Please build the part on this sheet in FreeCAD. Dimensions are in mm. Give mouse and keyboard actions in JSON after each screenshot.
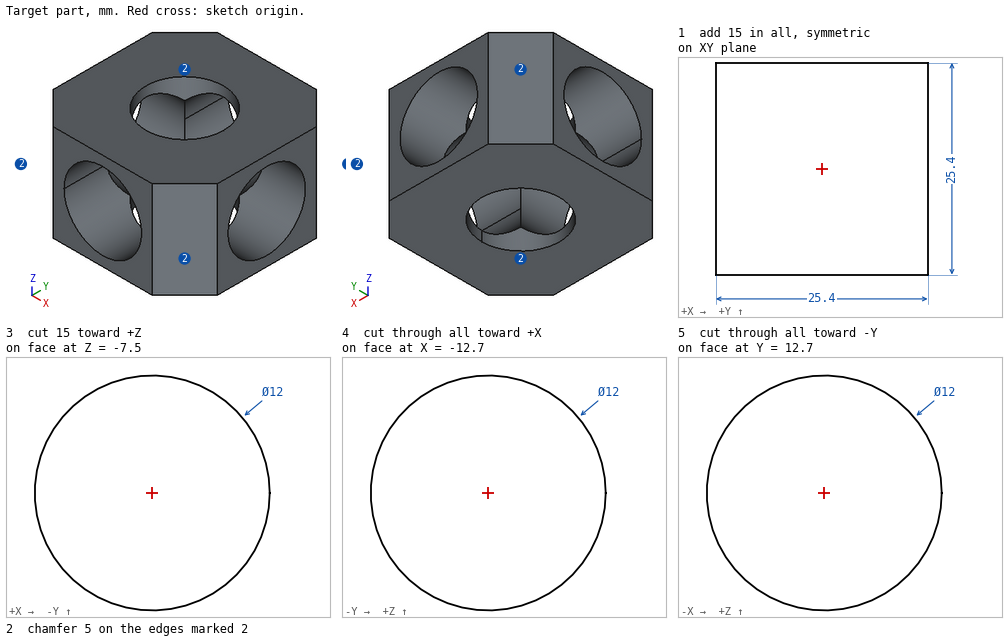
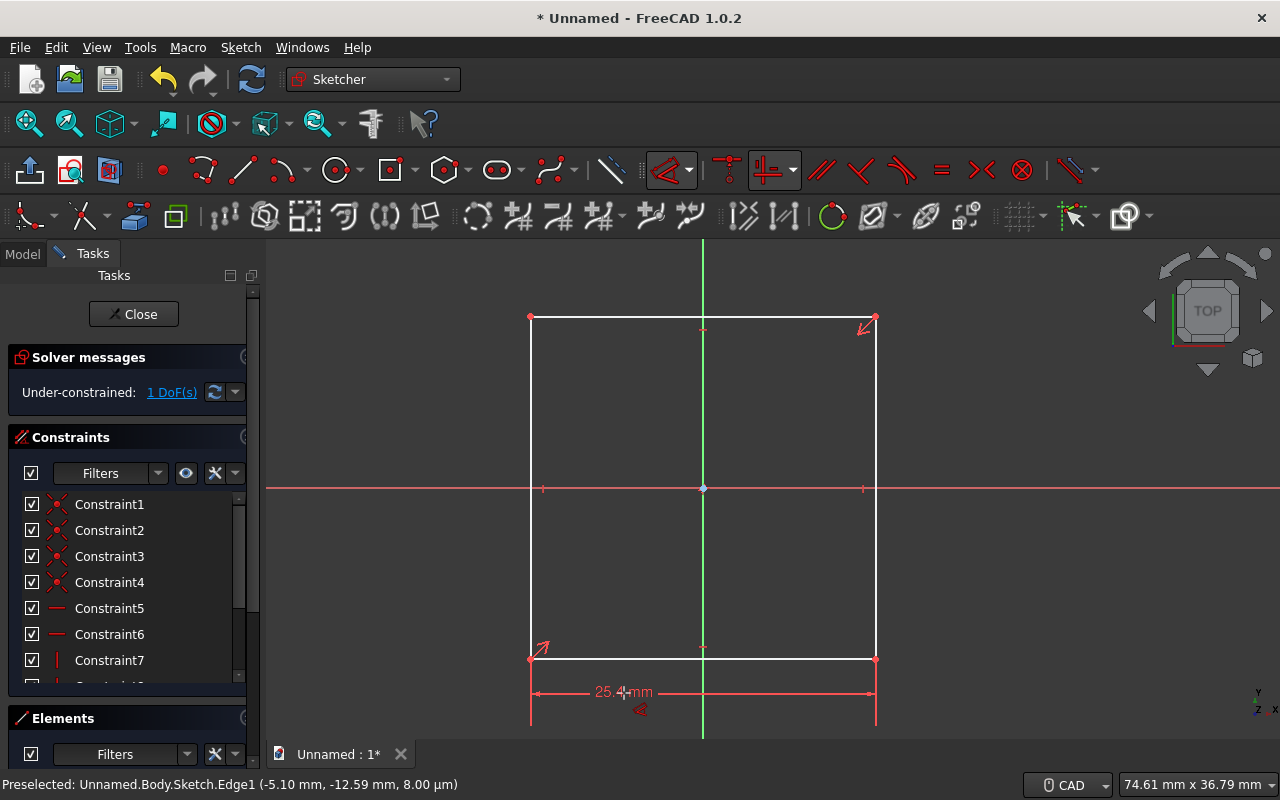
{"action": "left_click", "coordinate": [876, 557]}
{"action": "left_click", "coordinate": [910, 409]}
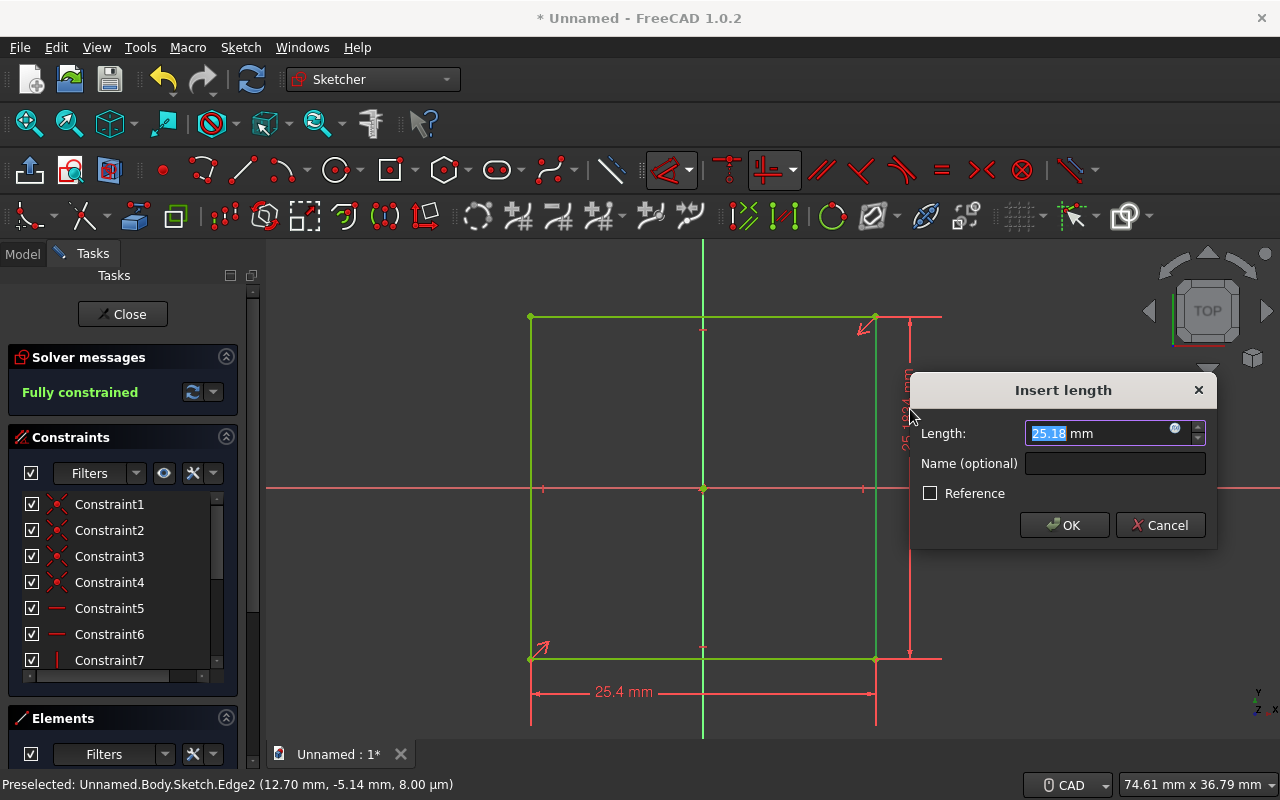
{"action": "type", "text": "25.4"}
{"action": "key", "text": "Return"}
{"action": "key", "text": "Escape"}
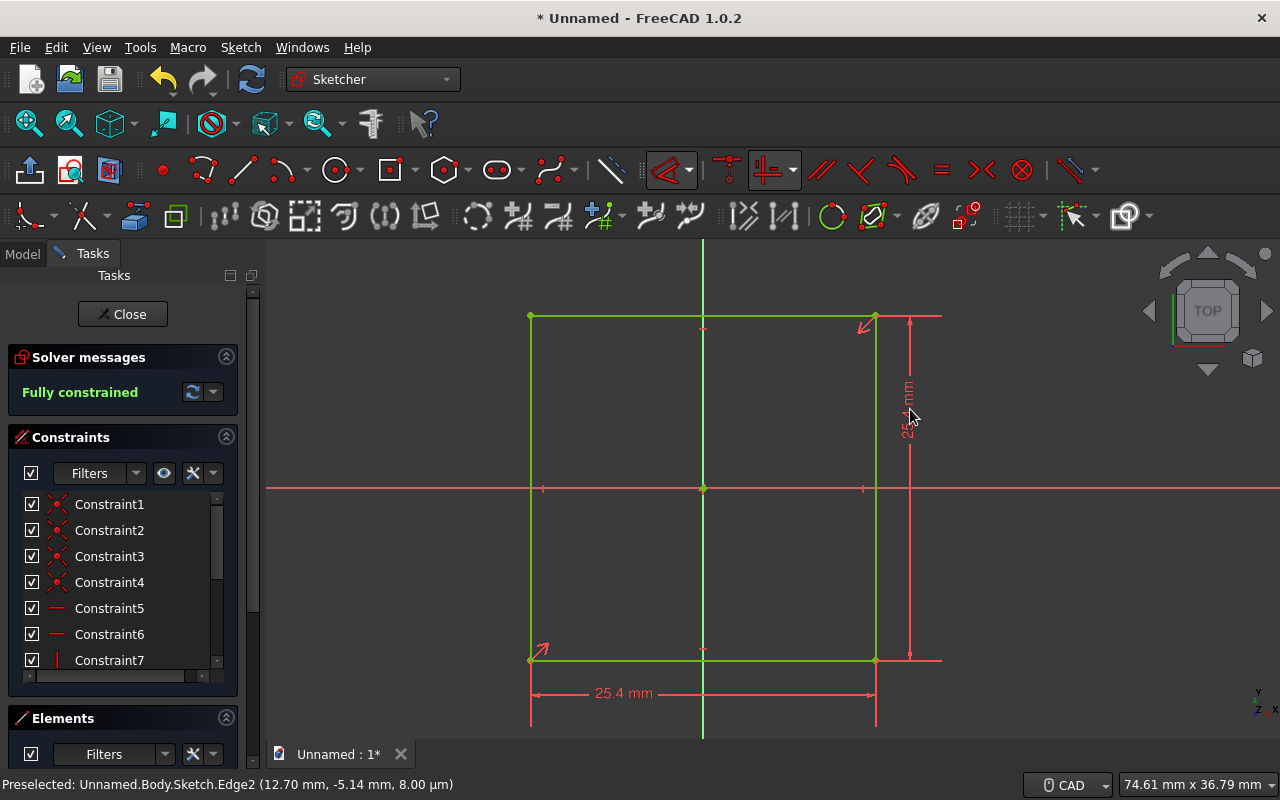
{"action": "left_click", "coordinate": [123, 314]}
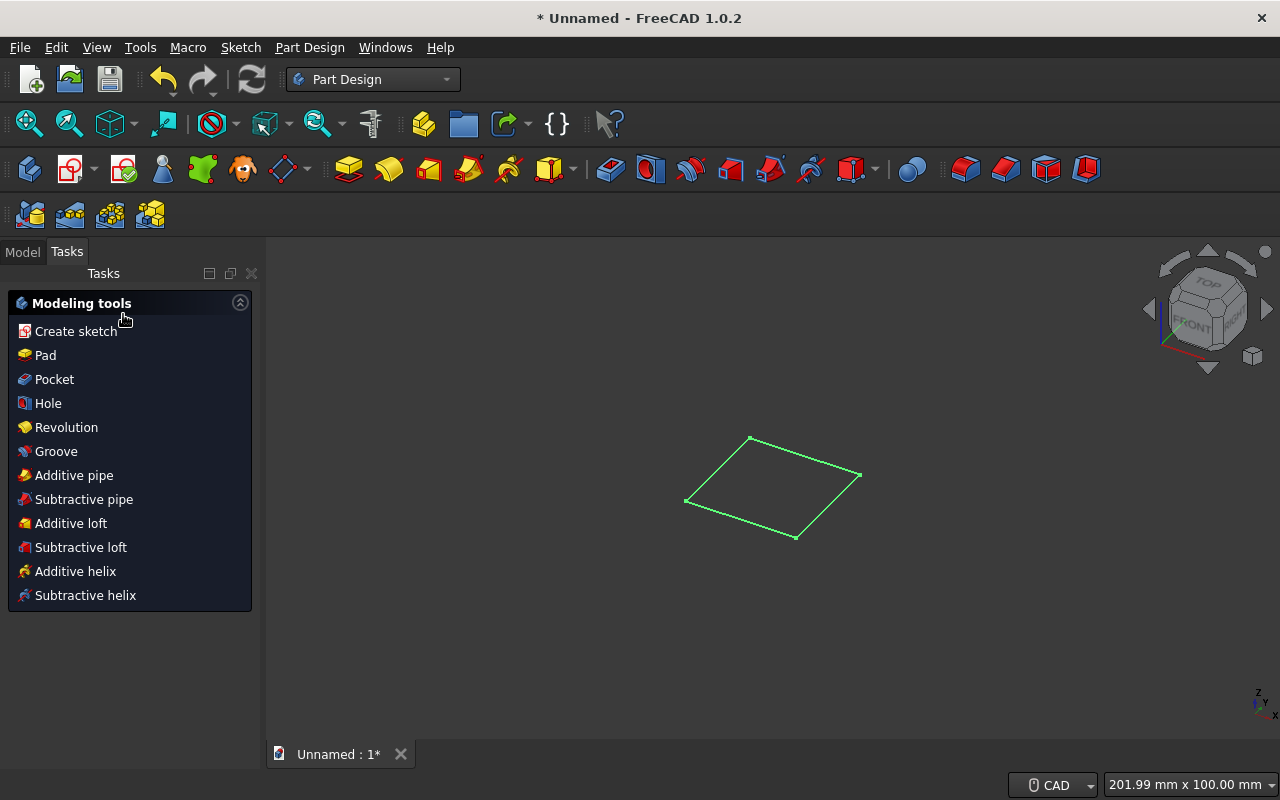
{"action": "left_click", "coordinate": [350, 170]}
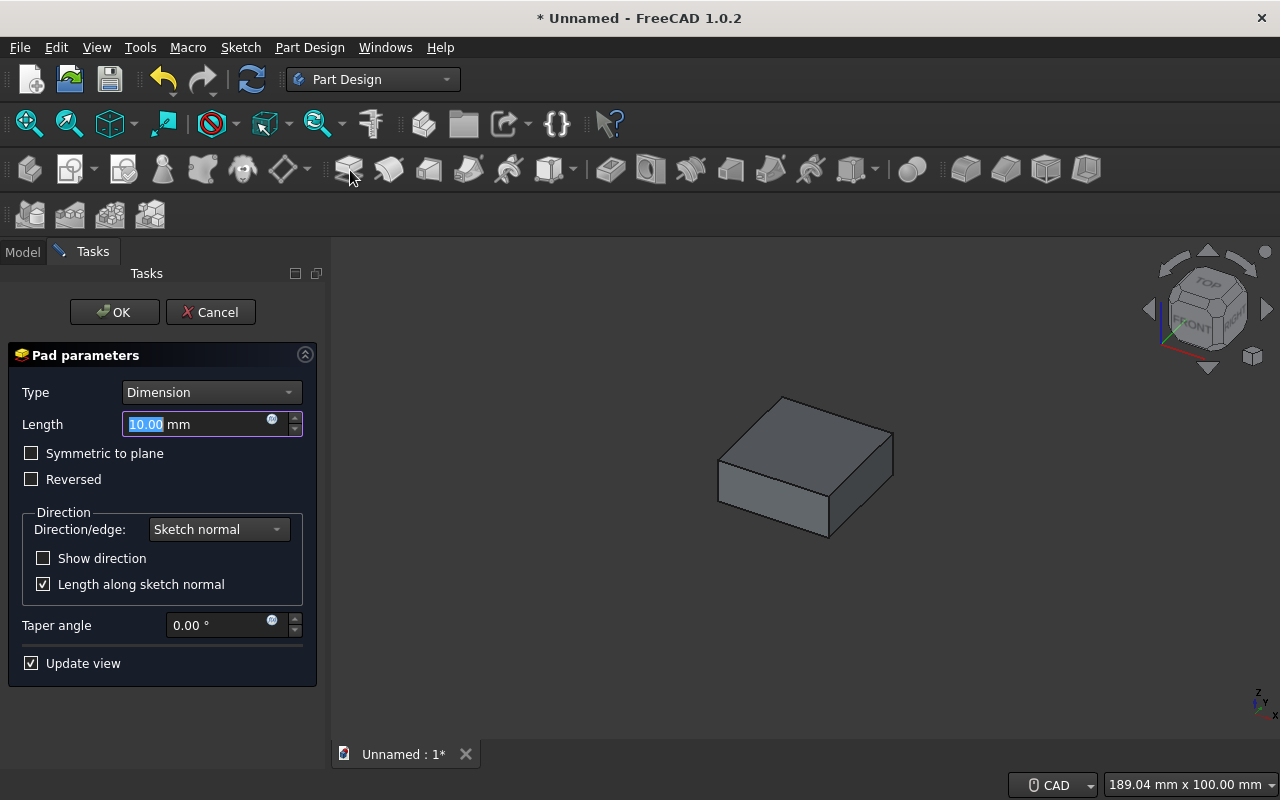
{"action": "type", "text": "15"}
{"action": "key", "text": "Tab"}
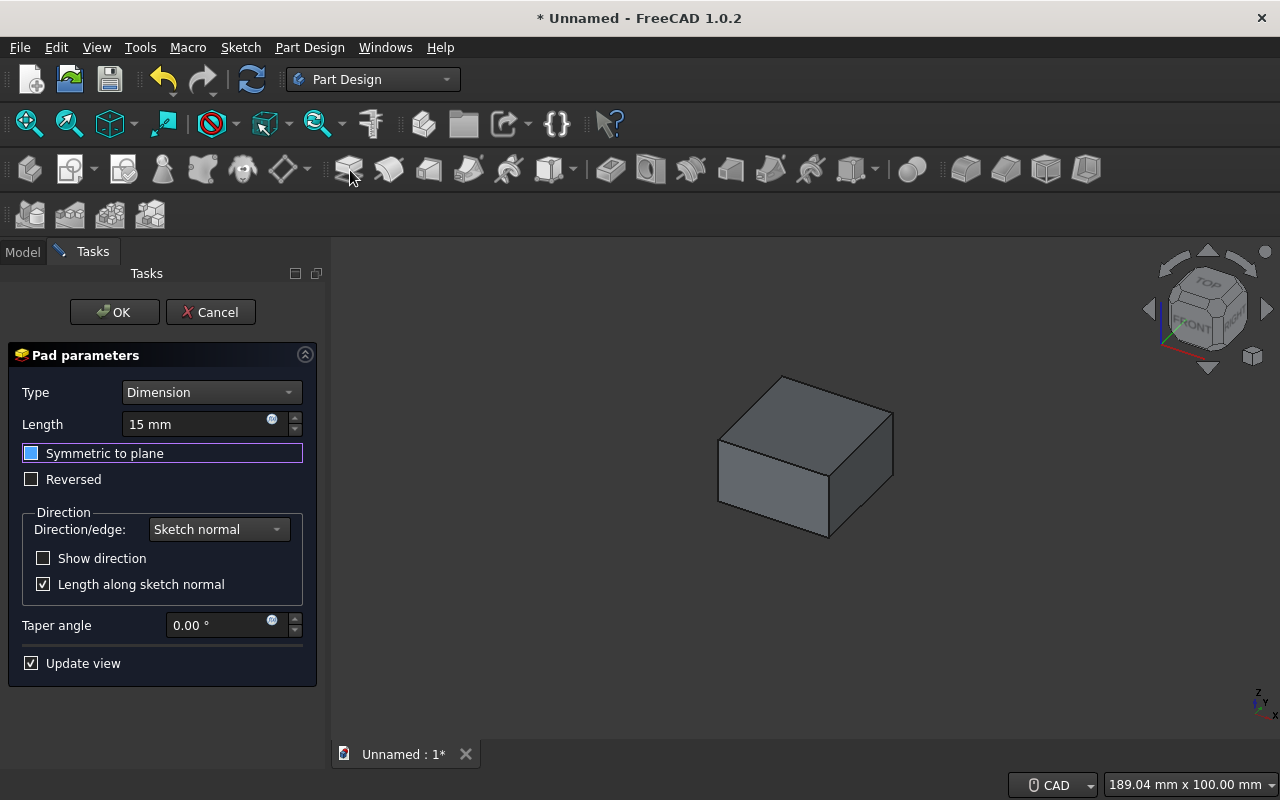
{"action": "left_click", "coordinate": [30, 453]}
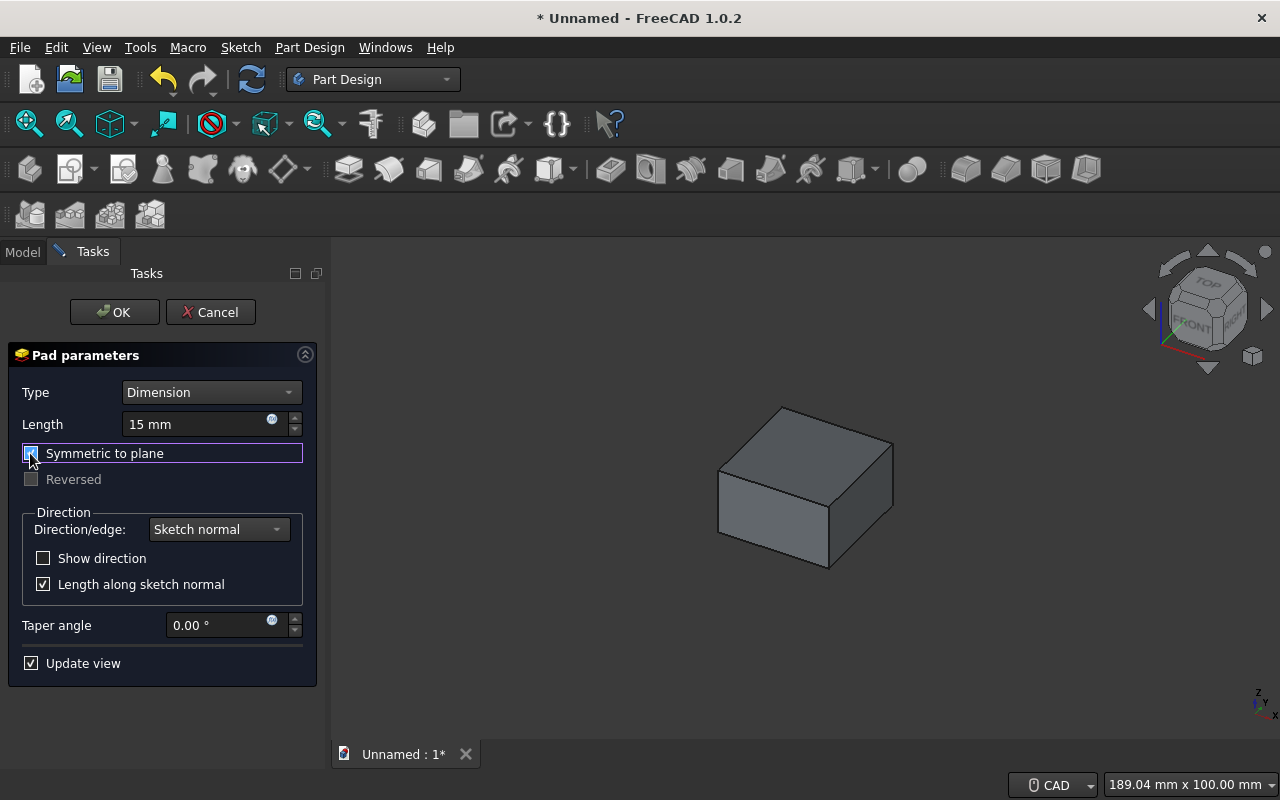
{"action": "left_click", "coordinate": [115, 312]}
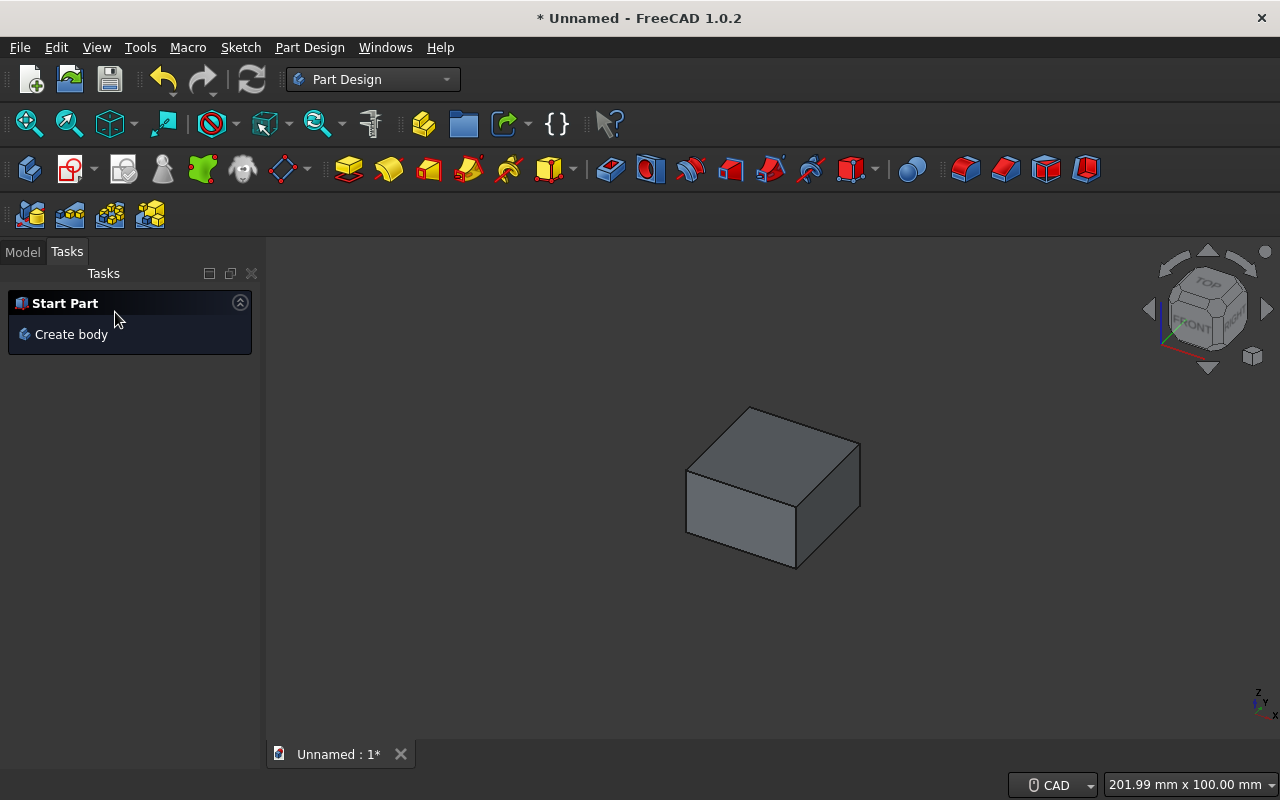
{"action": "key", "text": "v f"}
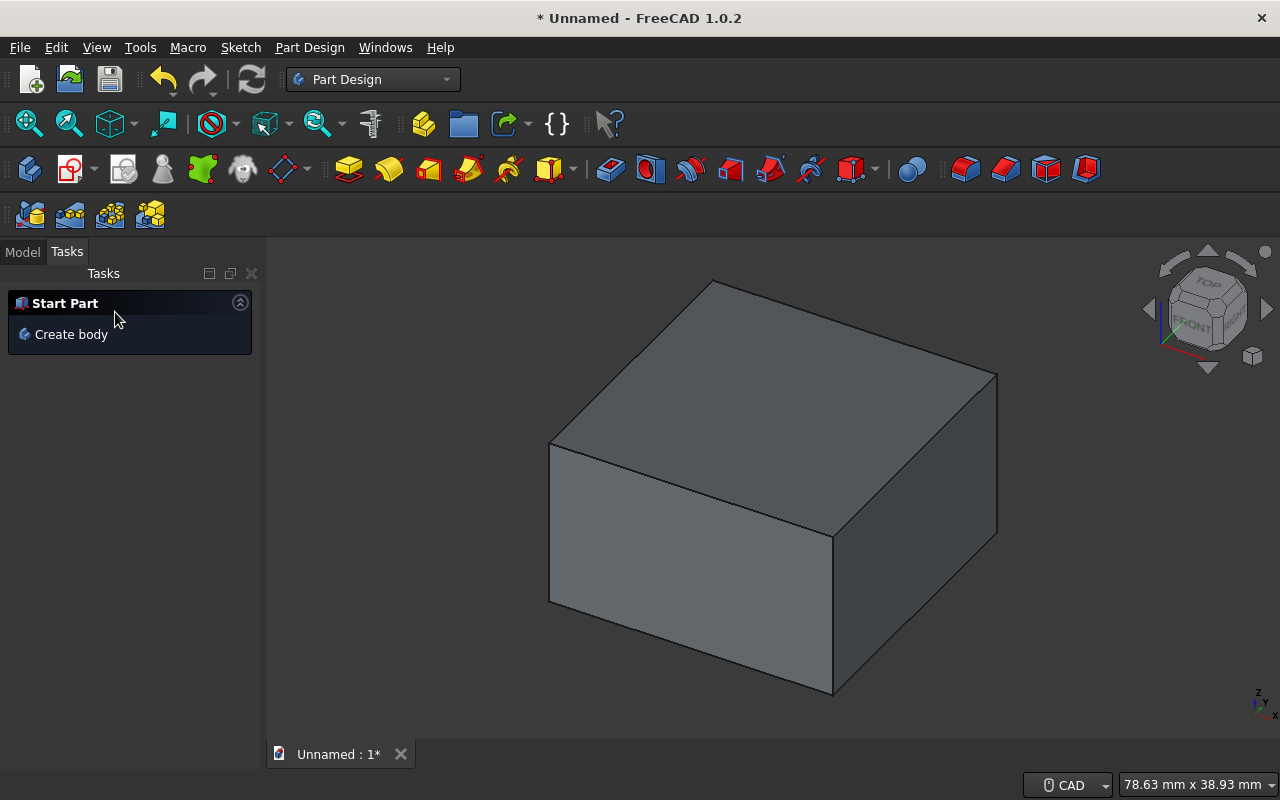
{"action": "left_click", "coordinate": [833, 615]}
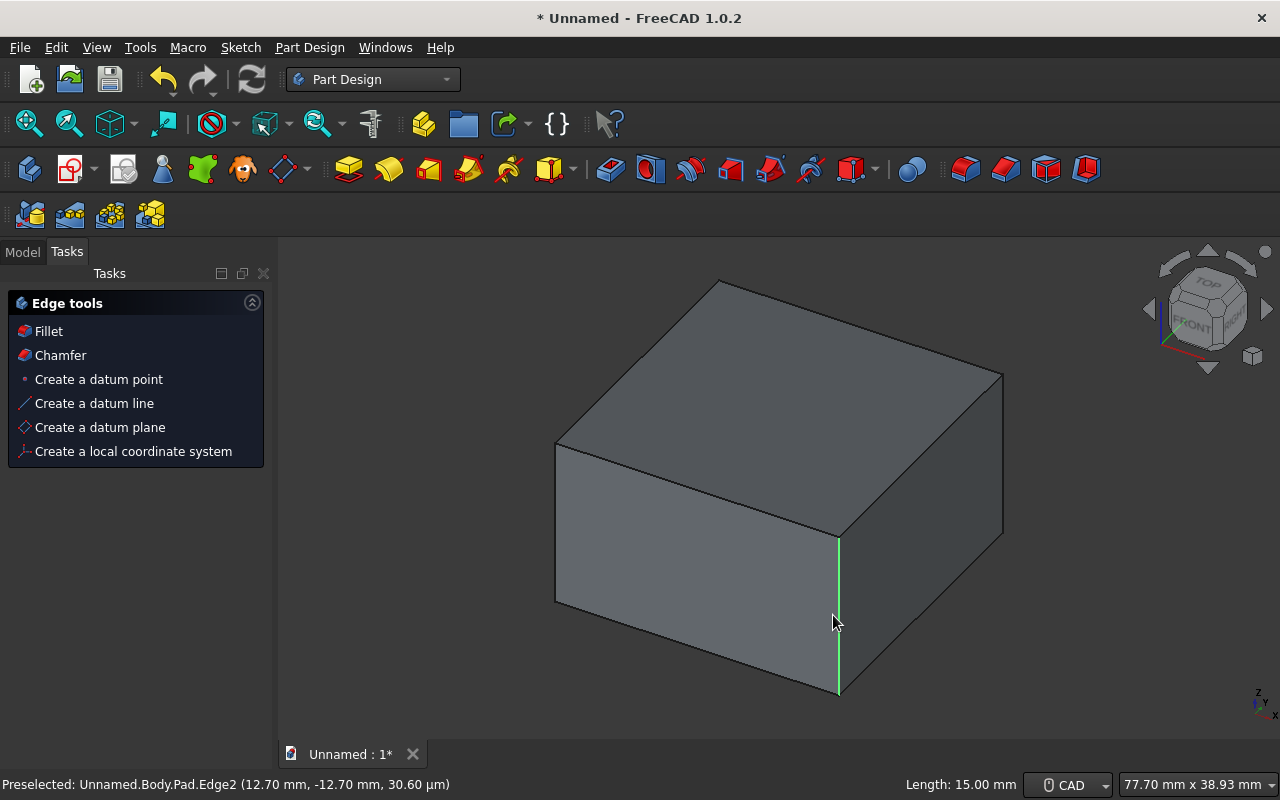
{"action": "key", "text": "0"}